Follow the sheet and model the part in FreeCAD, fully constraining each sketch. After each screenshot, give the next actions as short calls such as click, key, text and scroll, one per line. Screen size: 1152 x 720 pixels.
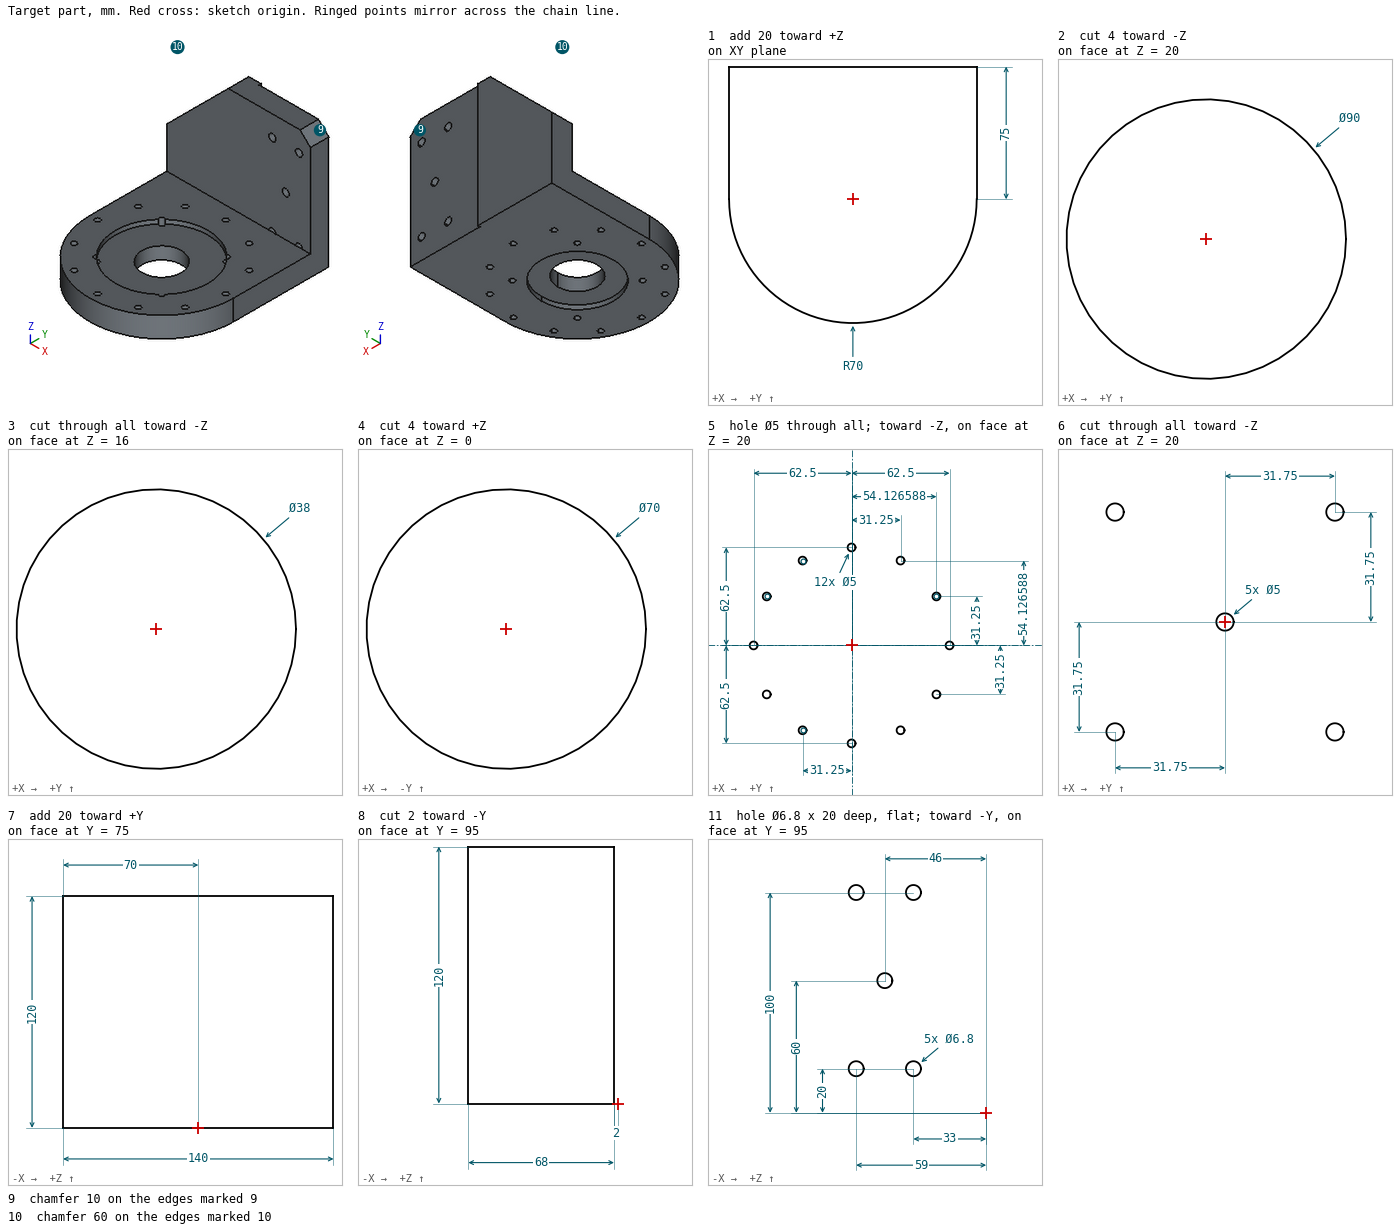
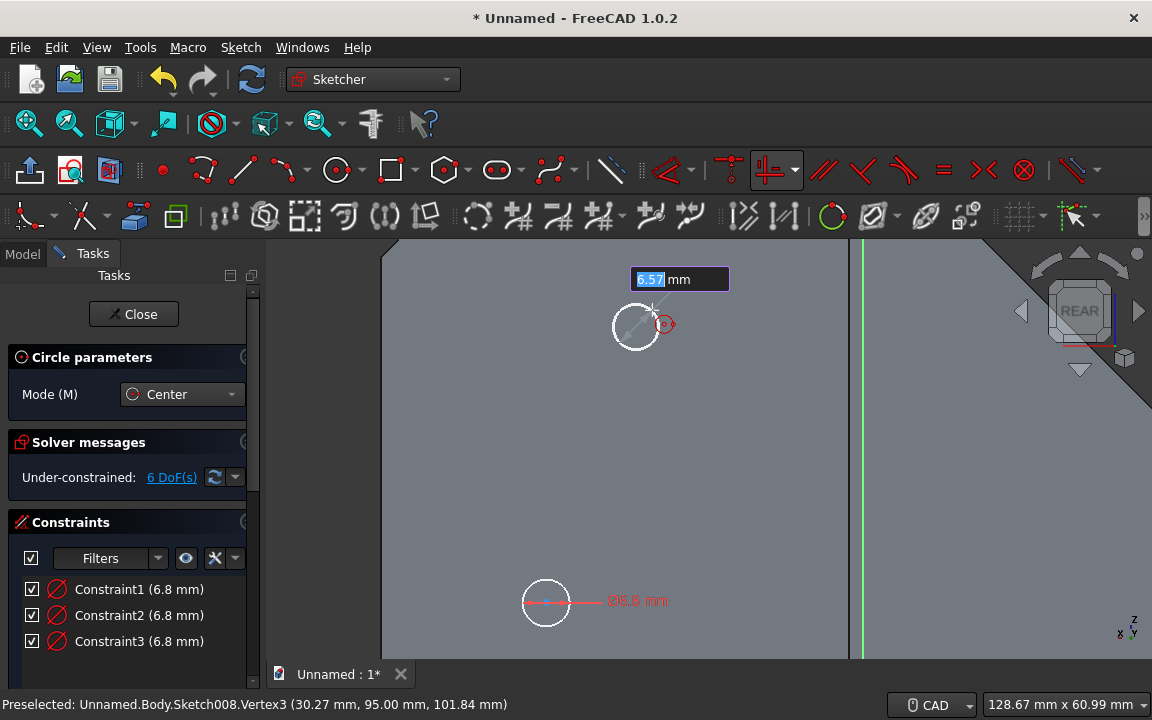
text(6.8)
key(Return)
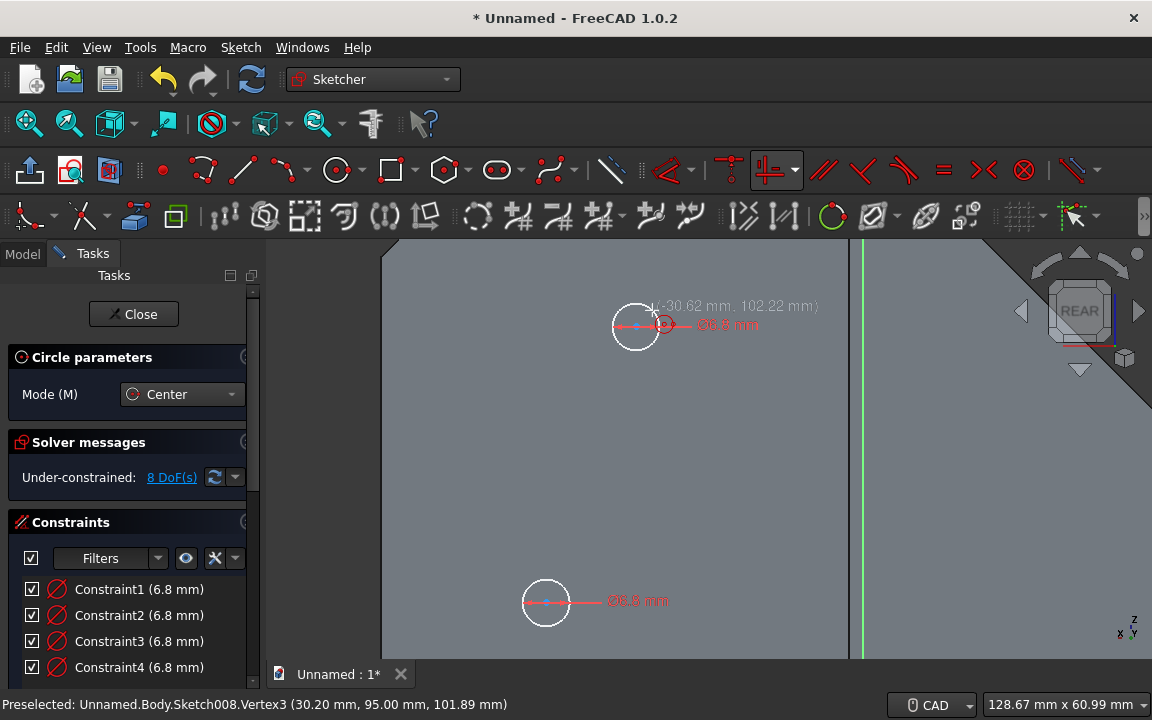
click(457, 326)
move(473, 310)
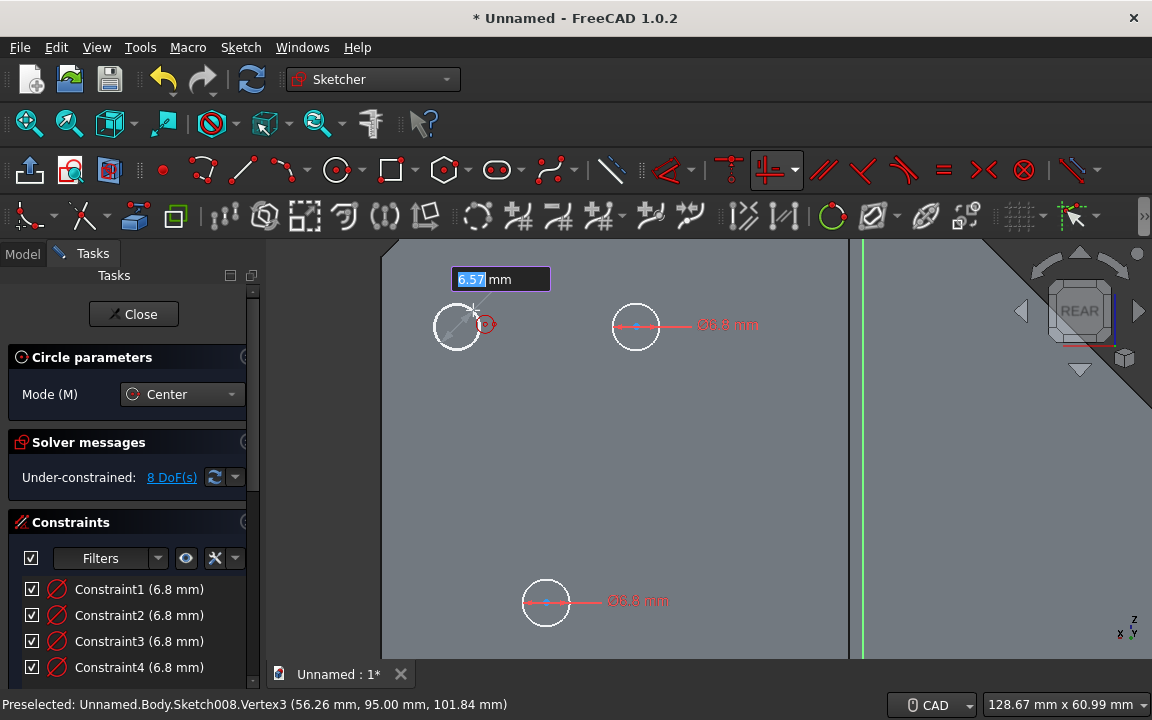
text(6.8)
key(Return)
key(Escape)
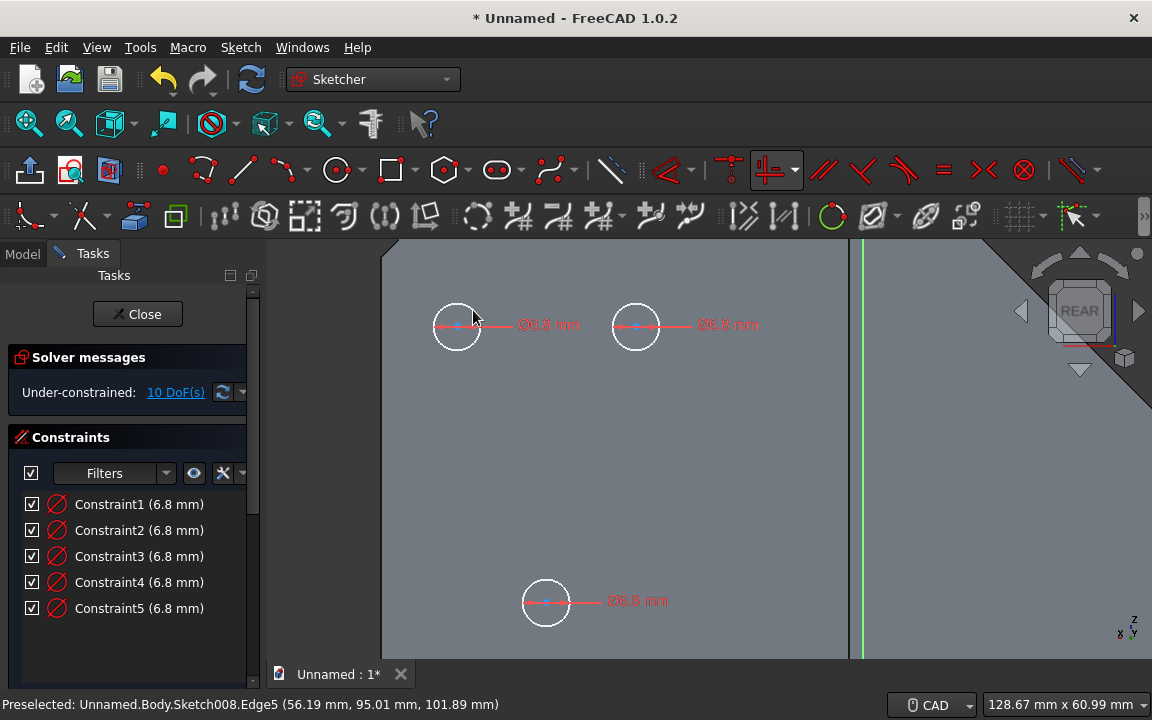
scroll(636, 327, down, 5)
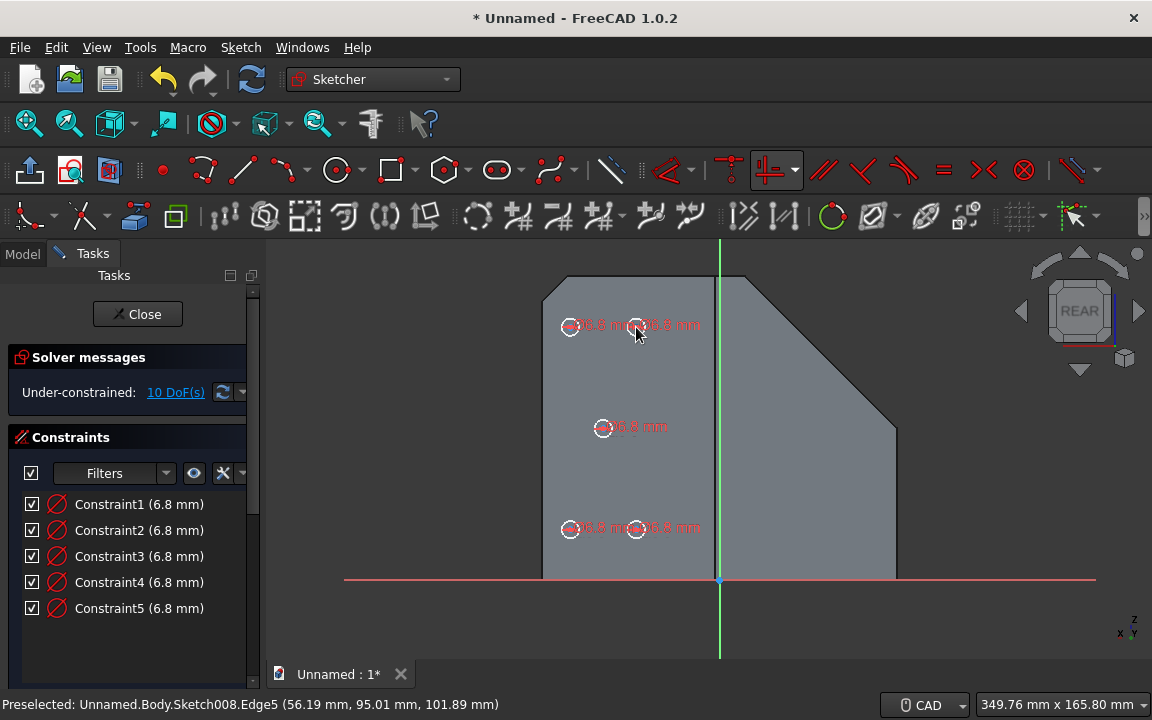
click(636, 530)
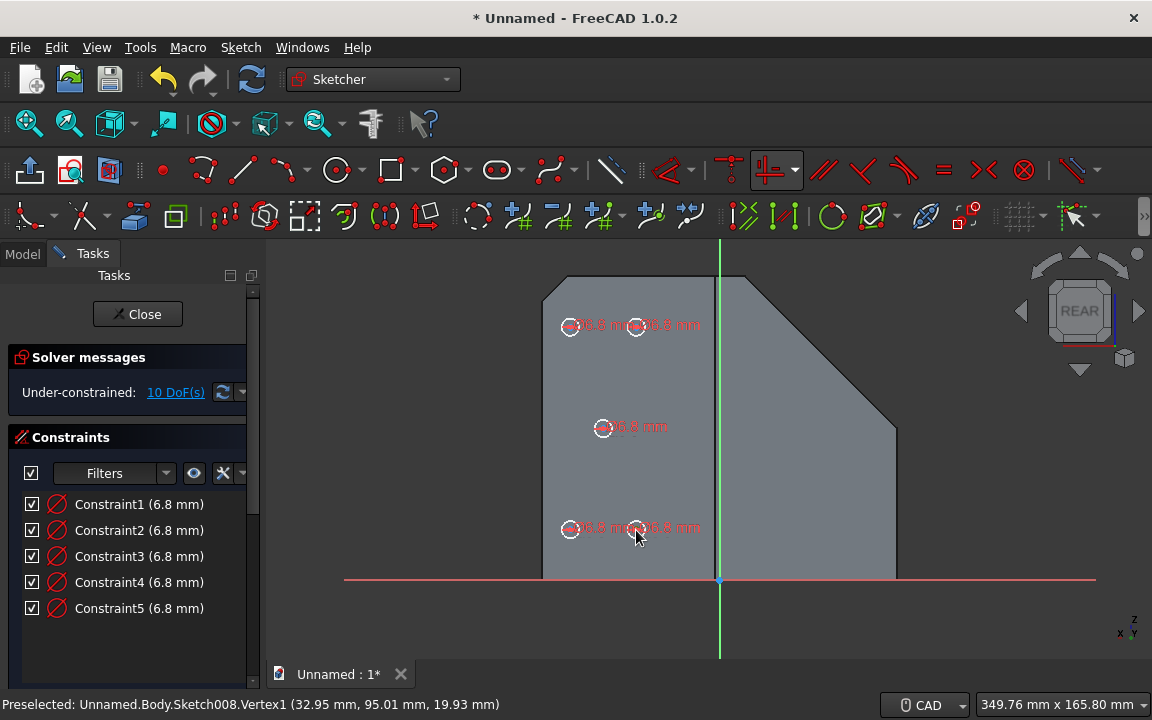
click(570, 530)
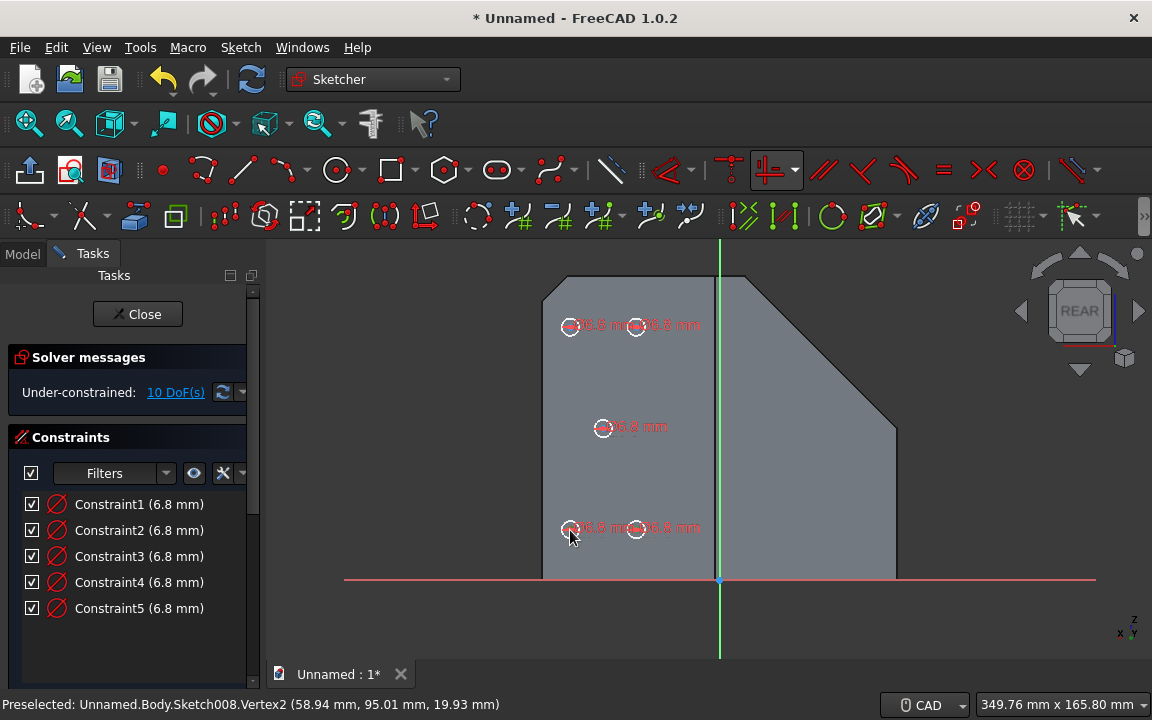
key(h)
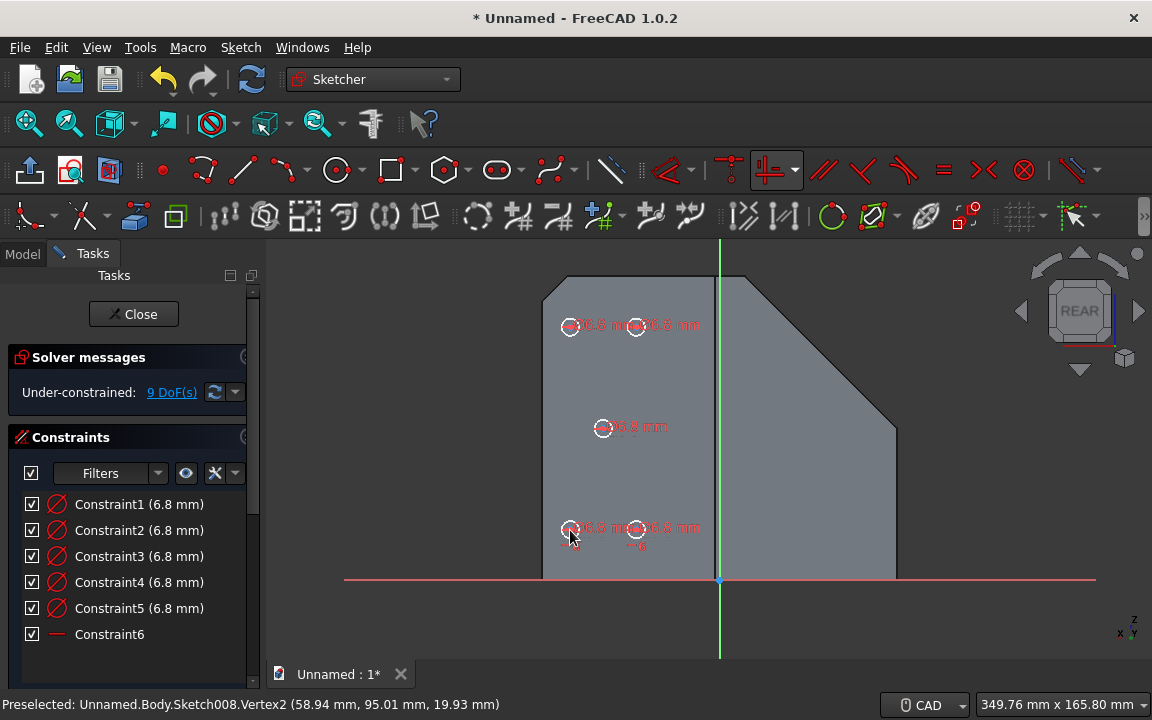
click(636, 530)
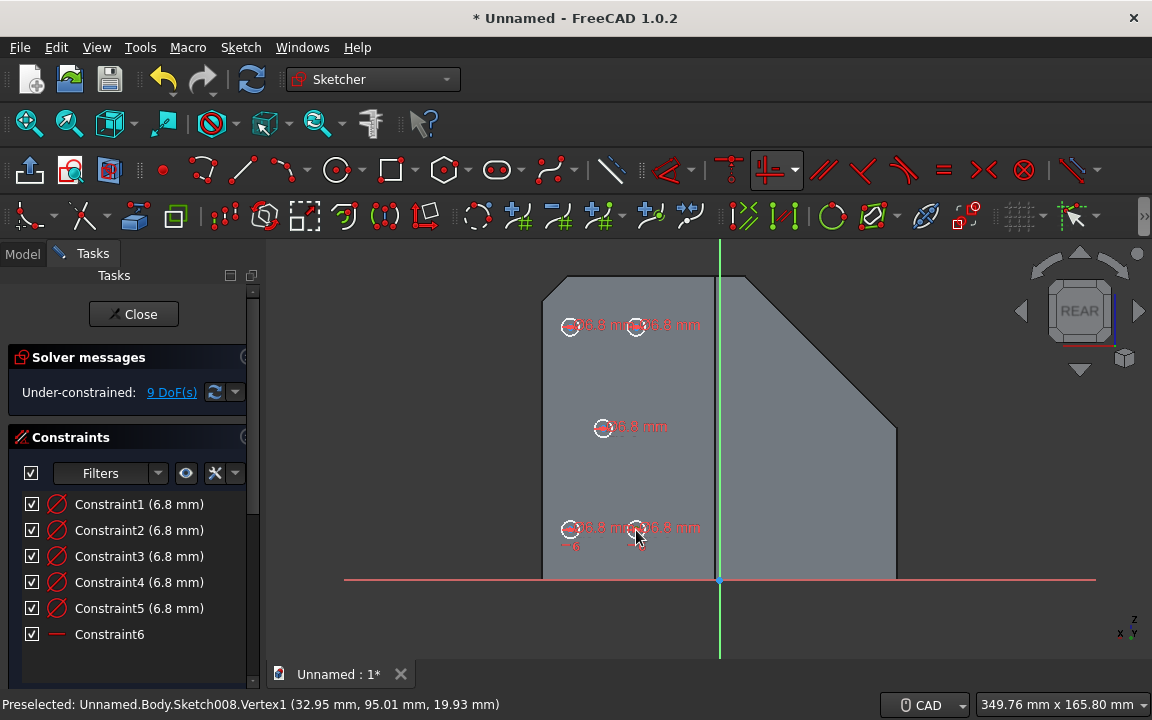
click(636, 327)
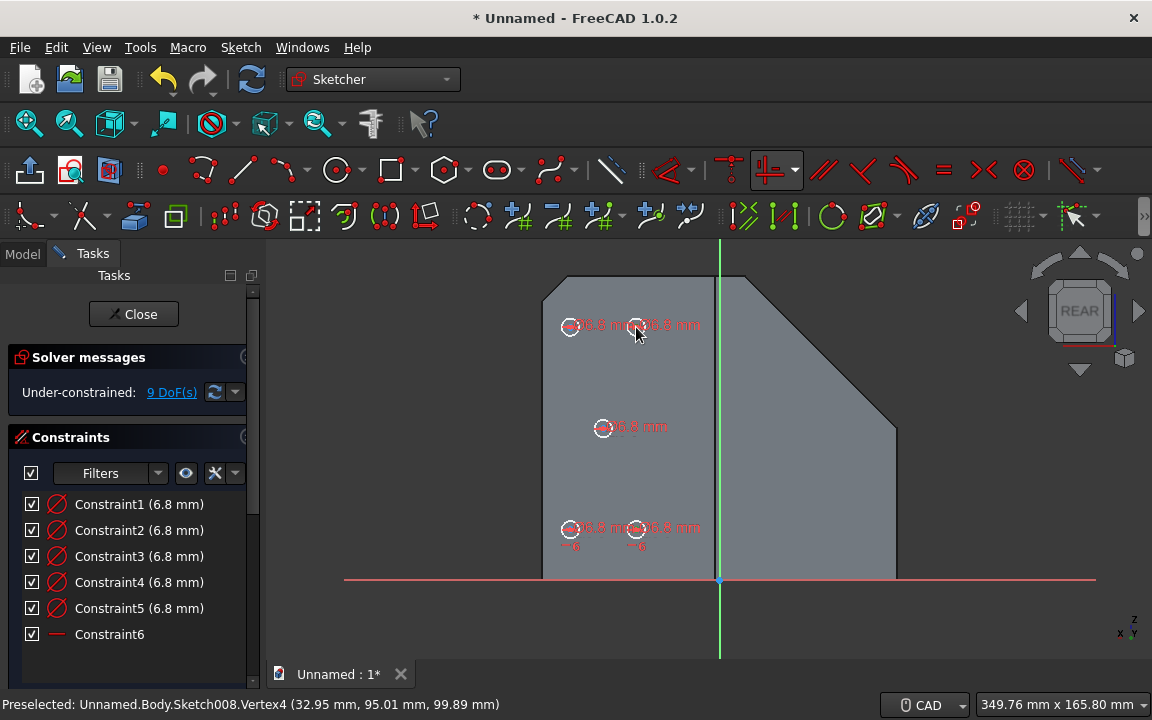
key(v)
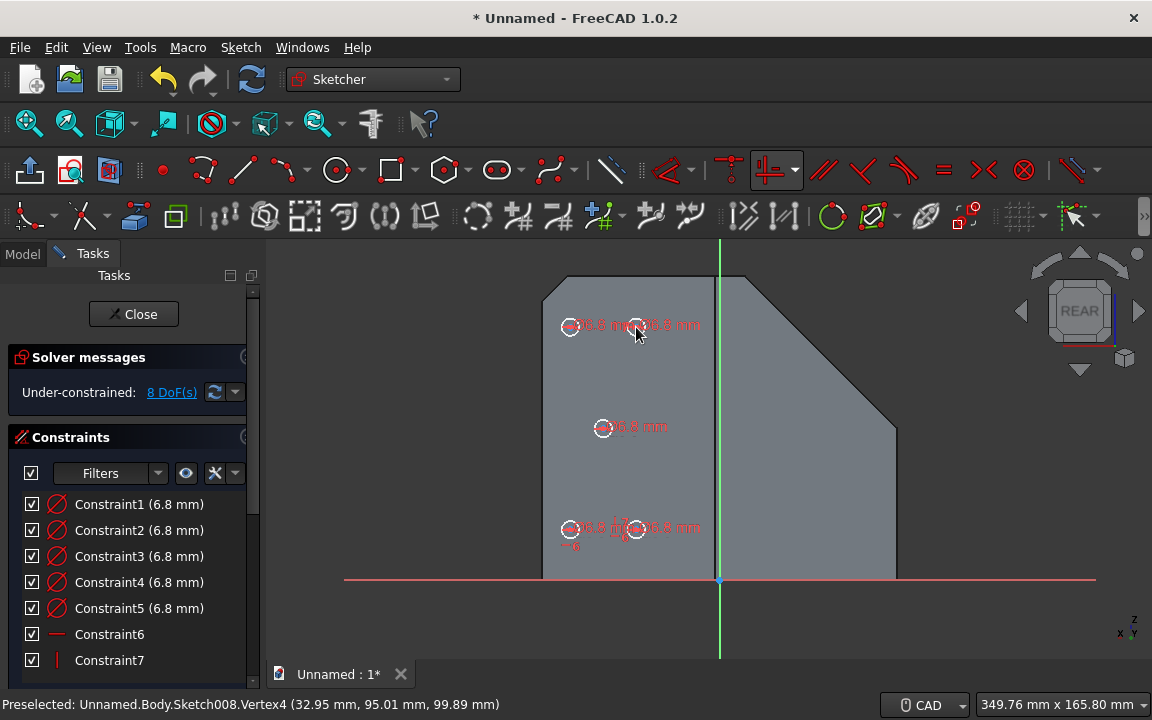
click(570, 530)